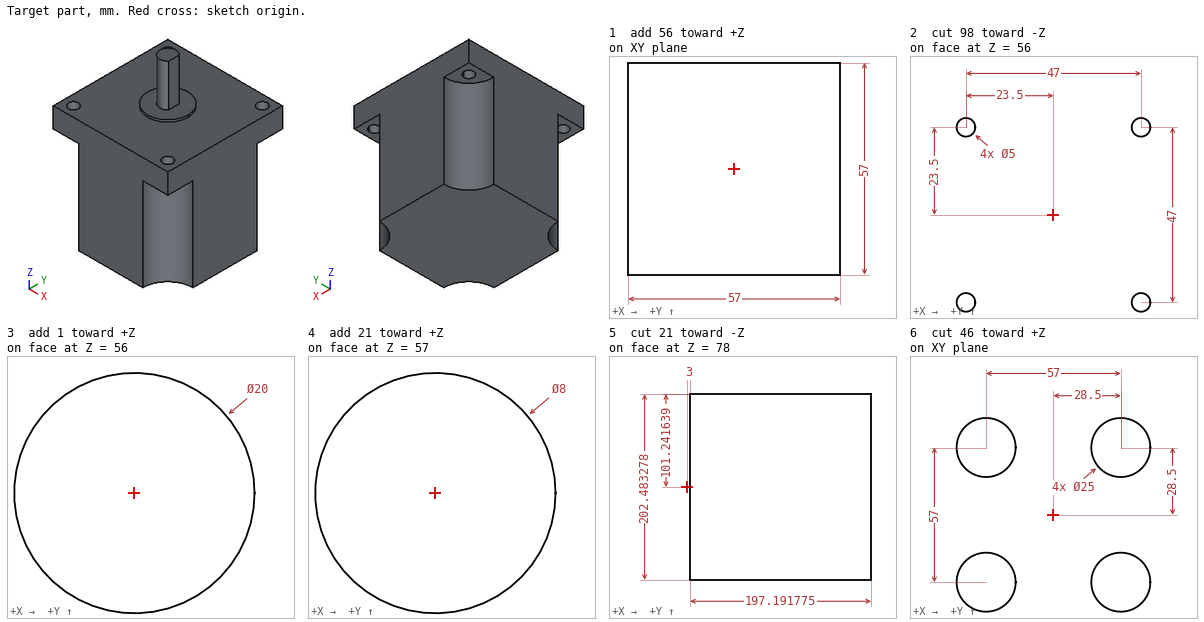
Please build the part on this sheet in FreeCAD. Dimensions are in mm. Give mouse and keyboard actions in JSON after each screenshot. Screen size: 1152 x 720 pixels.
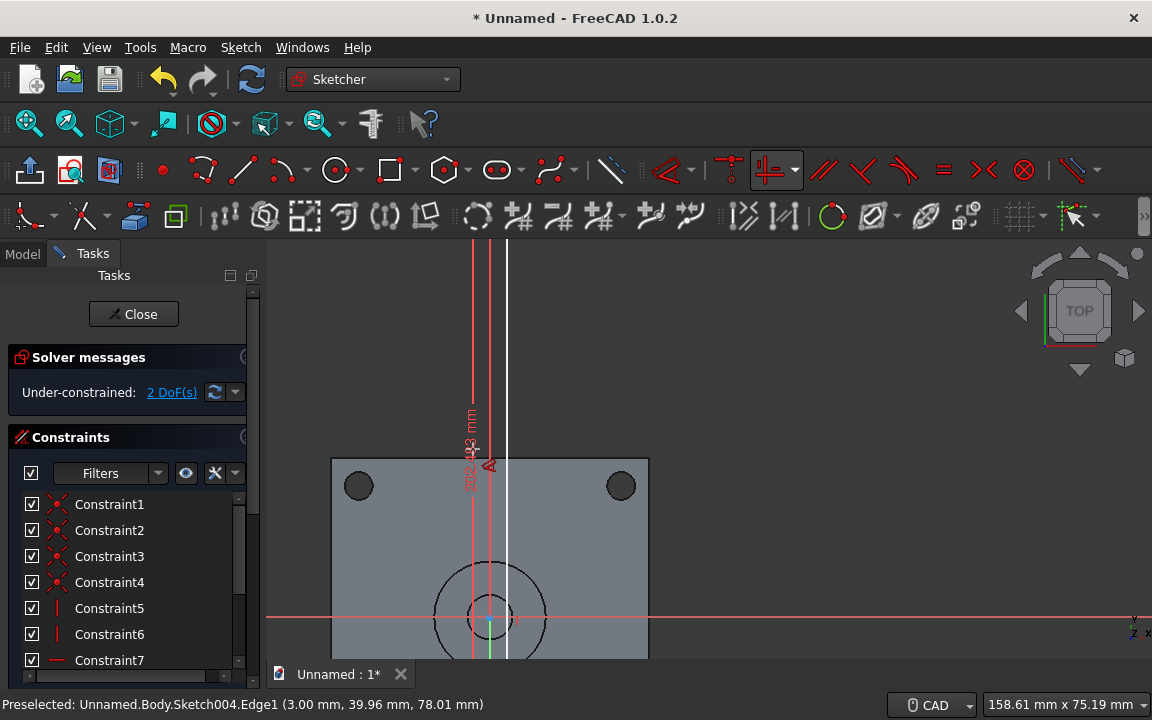
{"action": "scroll", "coordinate": [507, 394], "scroll_direction": "down", "scroll_amount": 7}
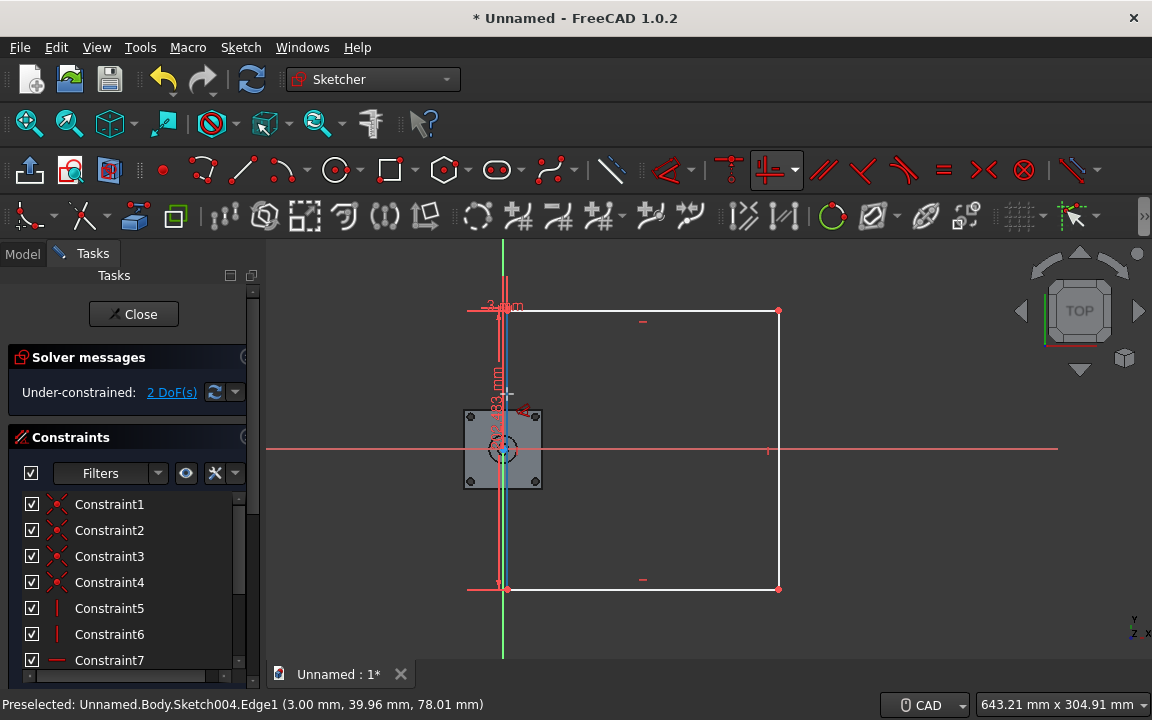
{"action": "left_click", "coordinate": [589, 590]}
{"action": "left_click", "coordinate": [643, 624]}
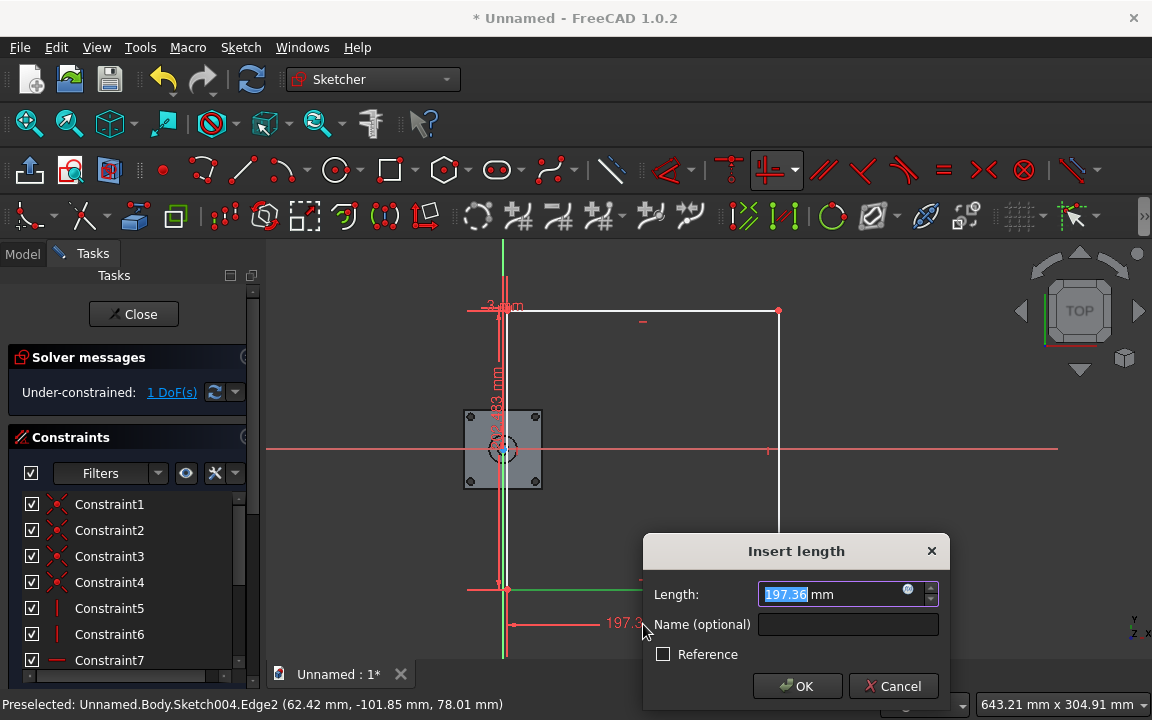
{"action": "type", "text": "197.191775"}
{"action": "key", "text": "Return"}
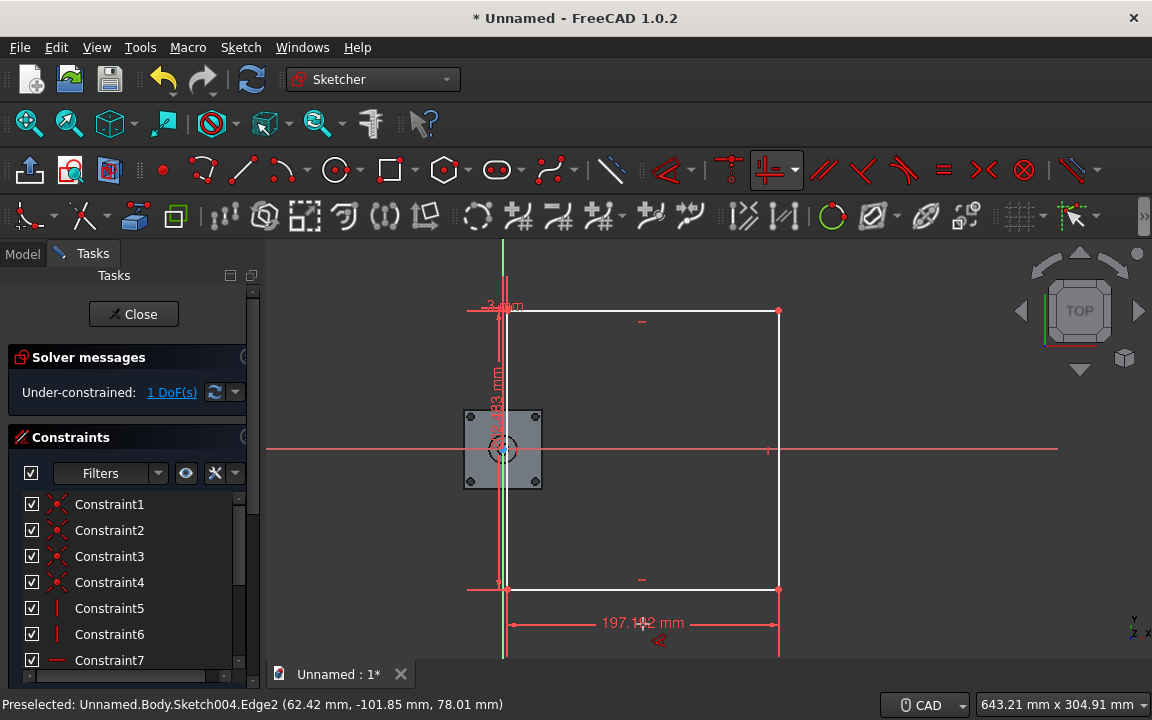
{"action": "left_click", "coordinate": [507, 311]}
{"action": "left_click", "coordinate": [469, 380]}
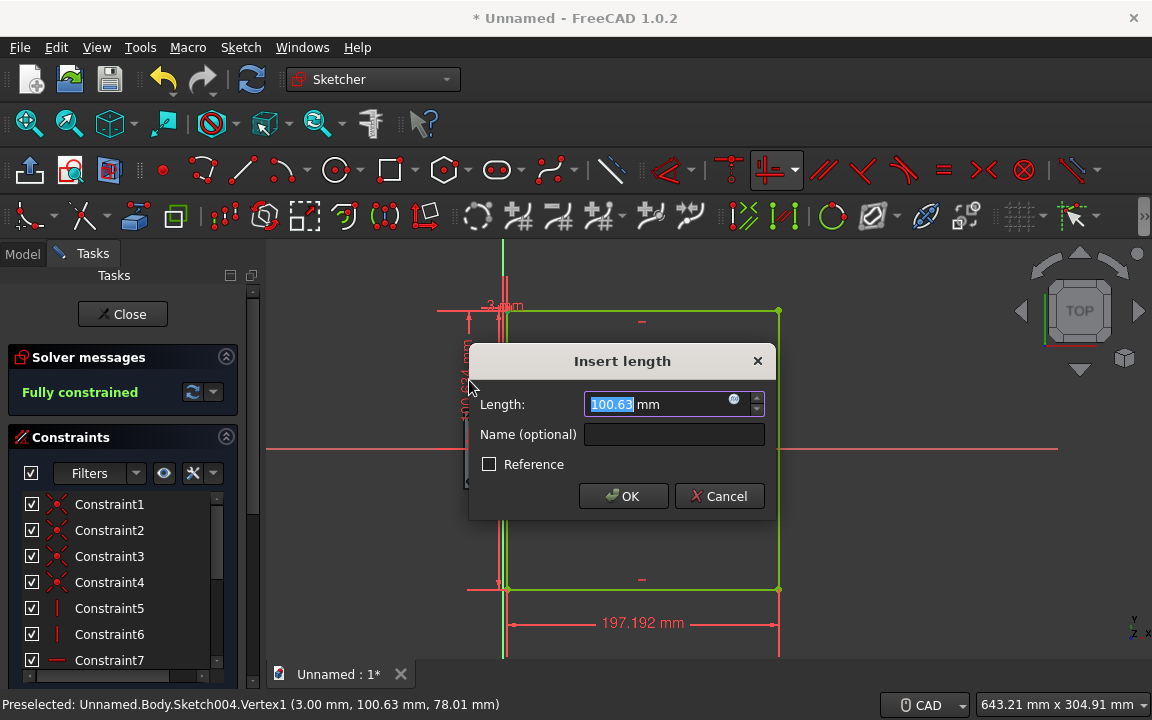
{"action": "type", "text": "101.241639"}
{"action": "key", "text": "Return"}
{"action": "key", "text": "Escape"}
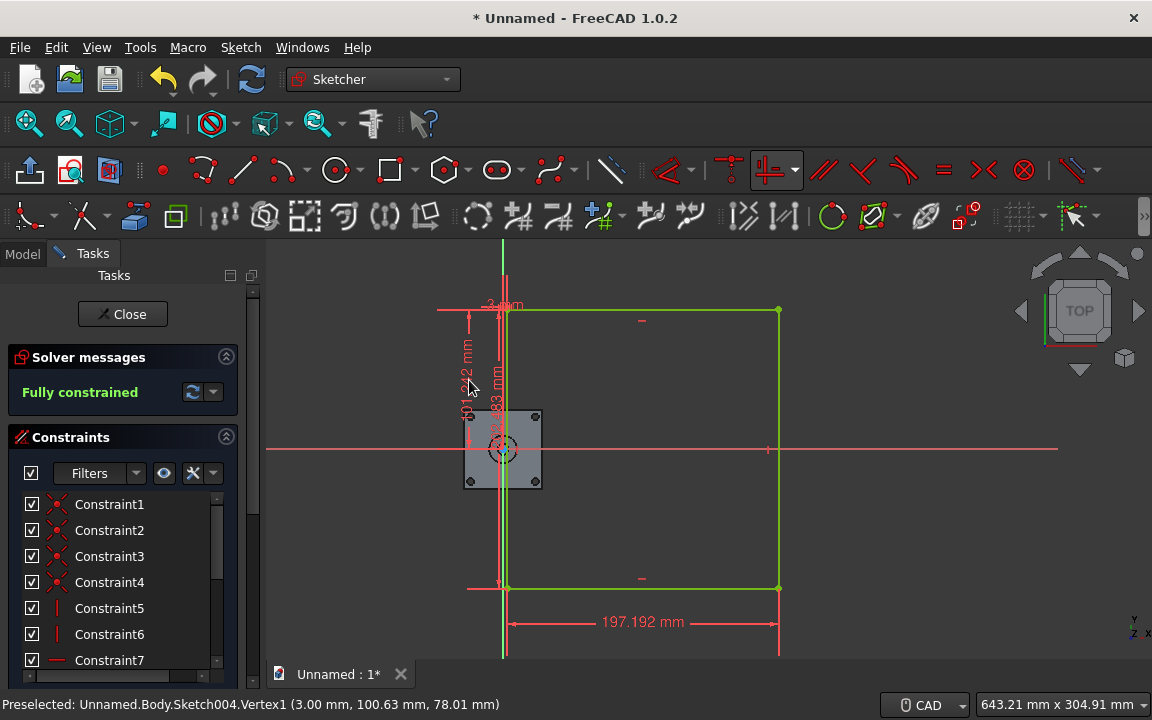
{"action": "left_click", "coordinate": [123, 314]}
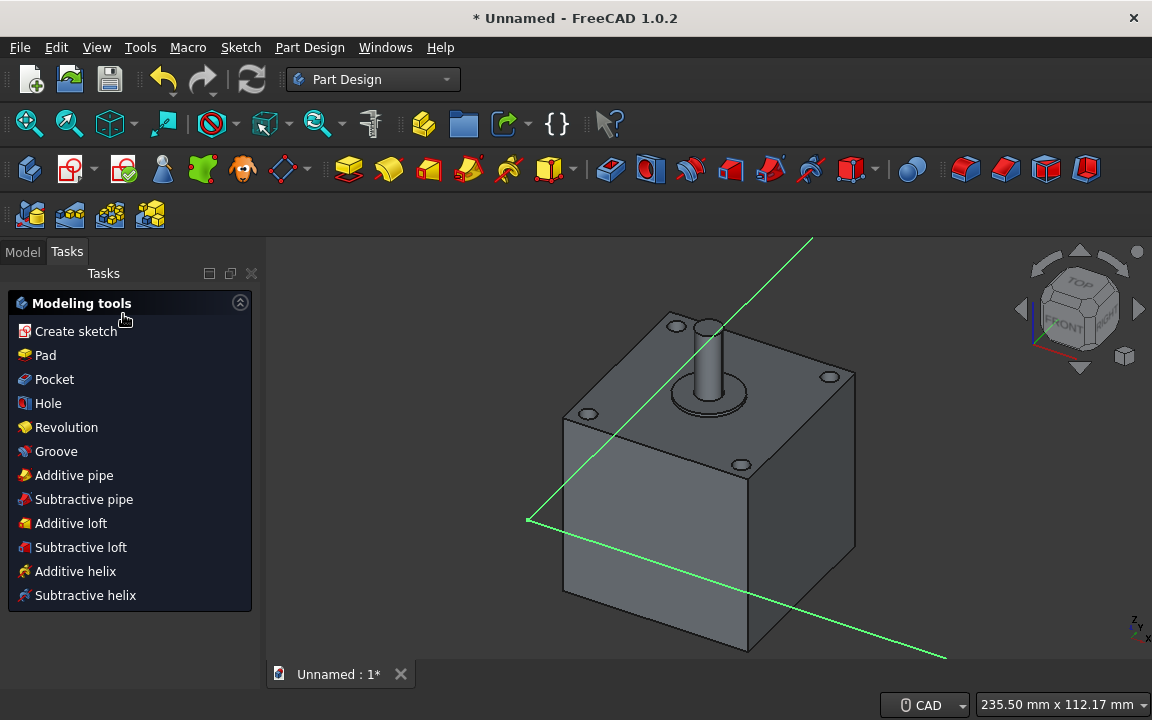
{"action": "left_click", "coordinate": [612, 170]}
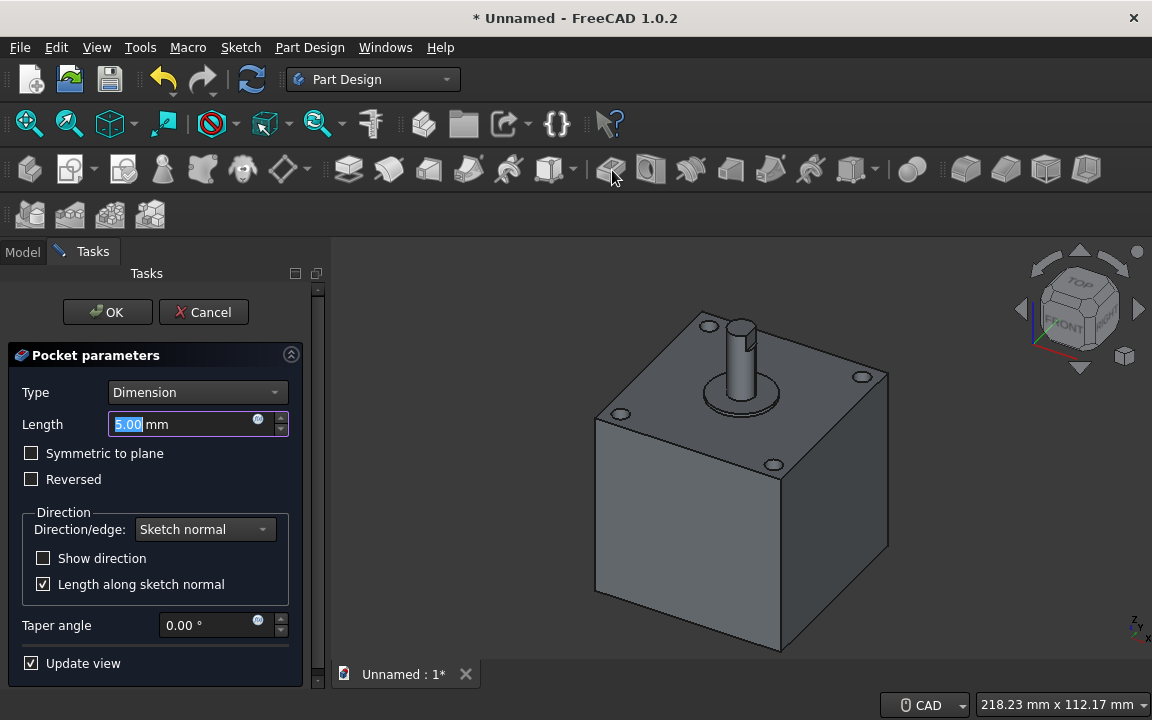
{"action": "type", "text": "21"}
{"action": "key", "text": "Tab"}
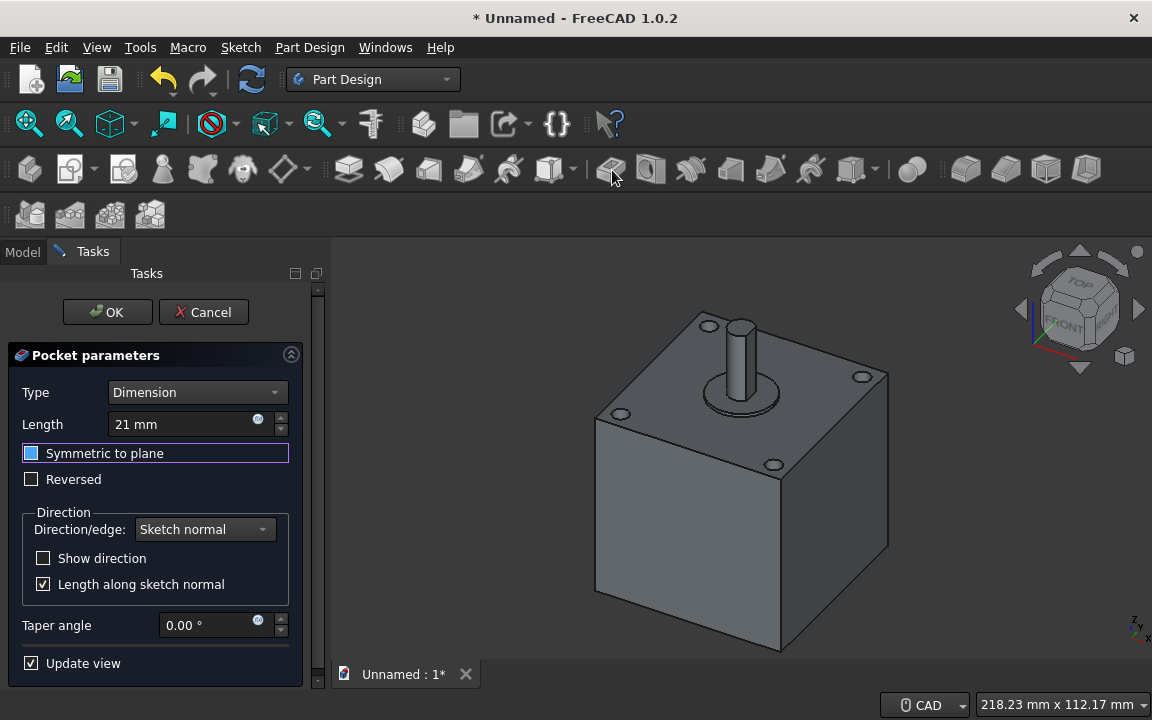
{"action": "left_click", "coordinate": [108, 312]}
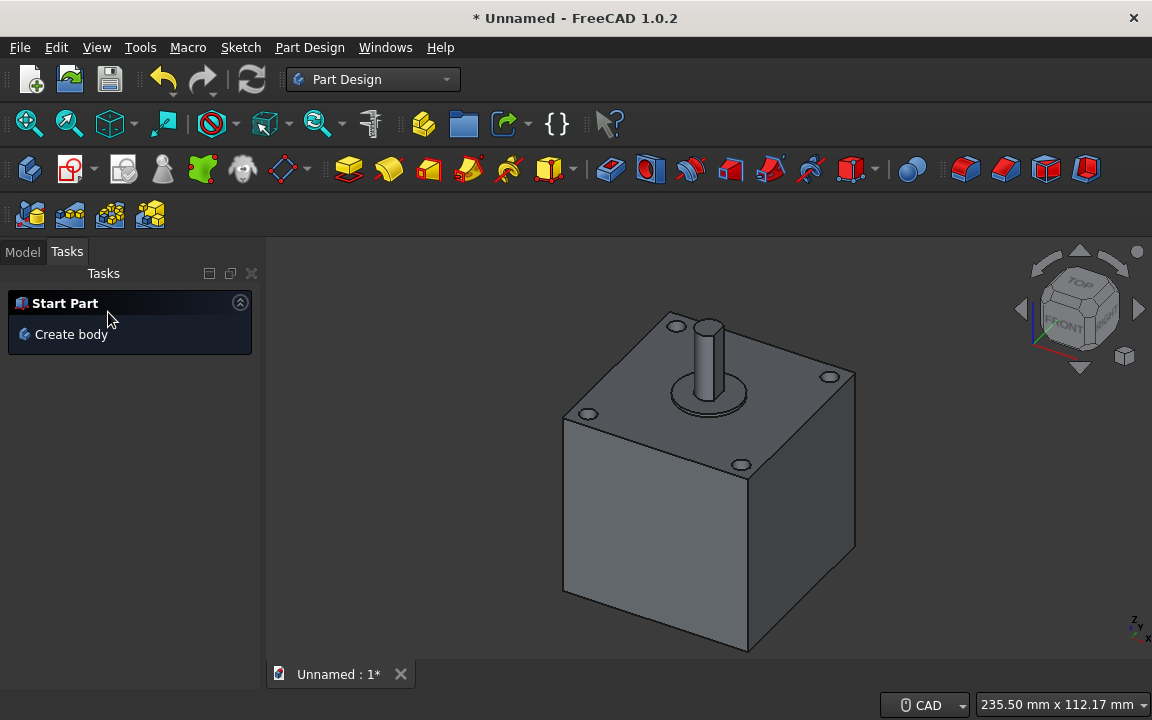
{"action": "left_click", "coordinate": [70, 170]}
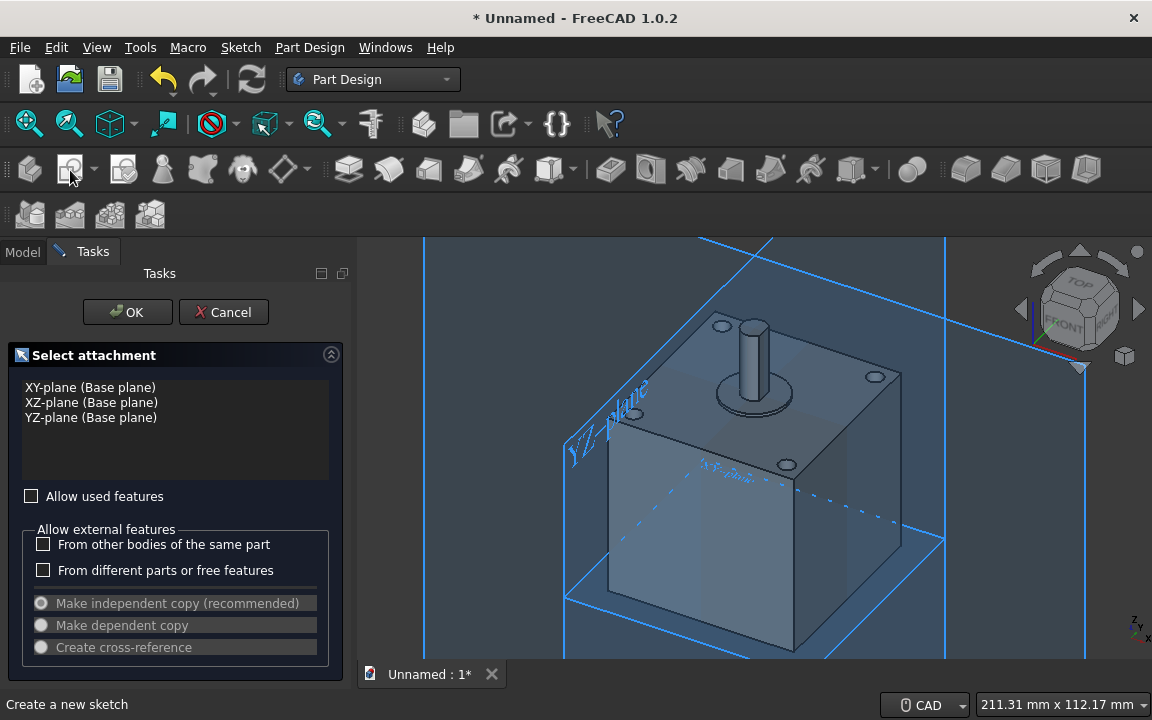
{"action": "left_click", "coordinate": [82, 388]}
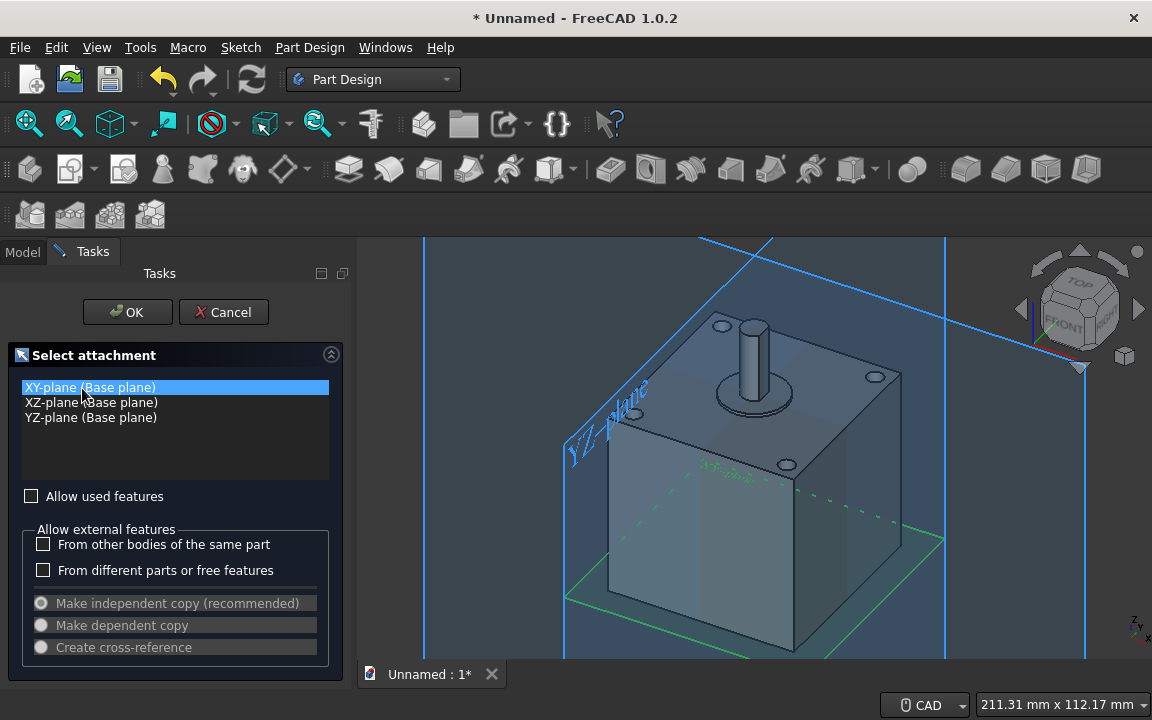
{"action": "left_click", "coordinate": [128, 312]}